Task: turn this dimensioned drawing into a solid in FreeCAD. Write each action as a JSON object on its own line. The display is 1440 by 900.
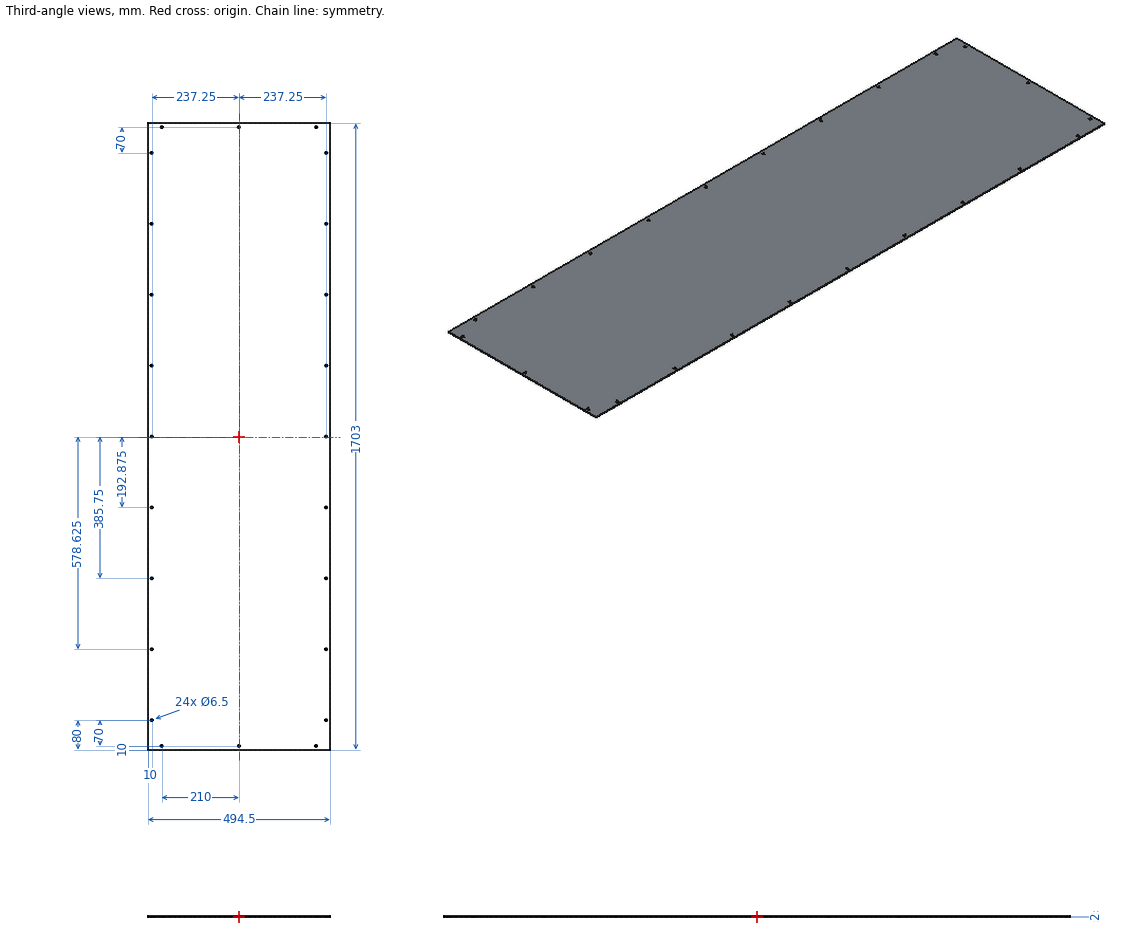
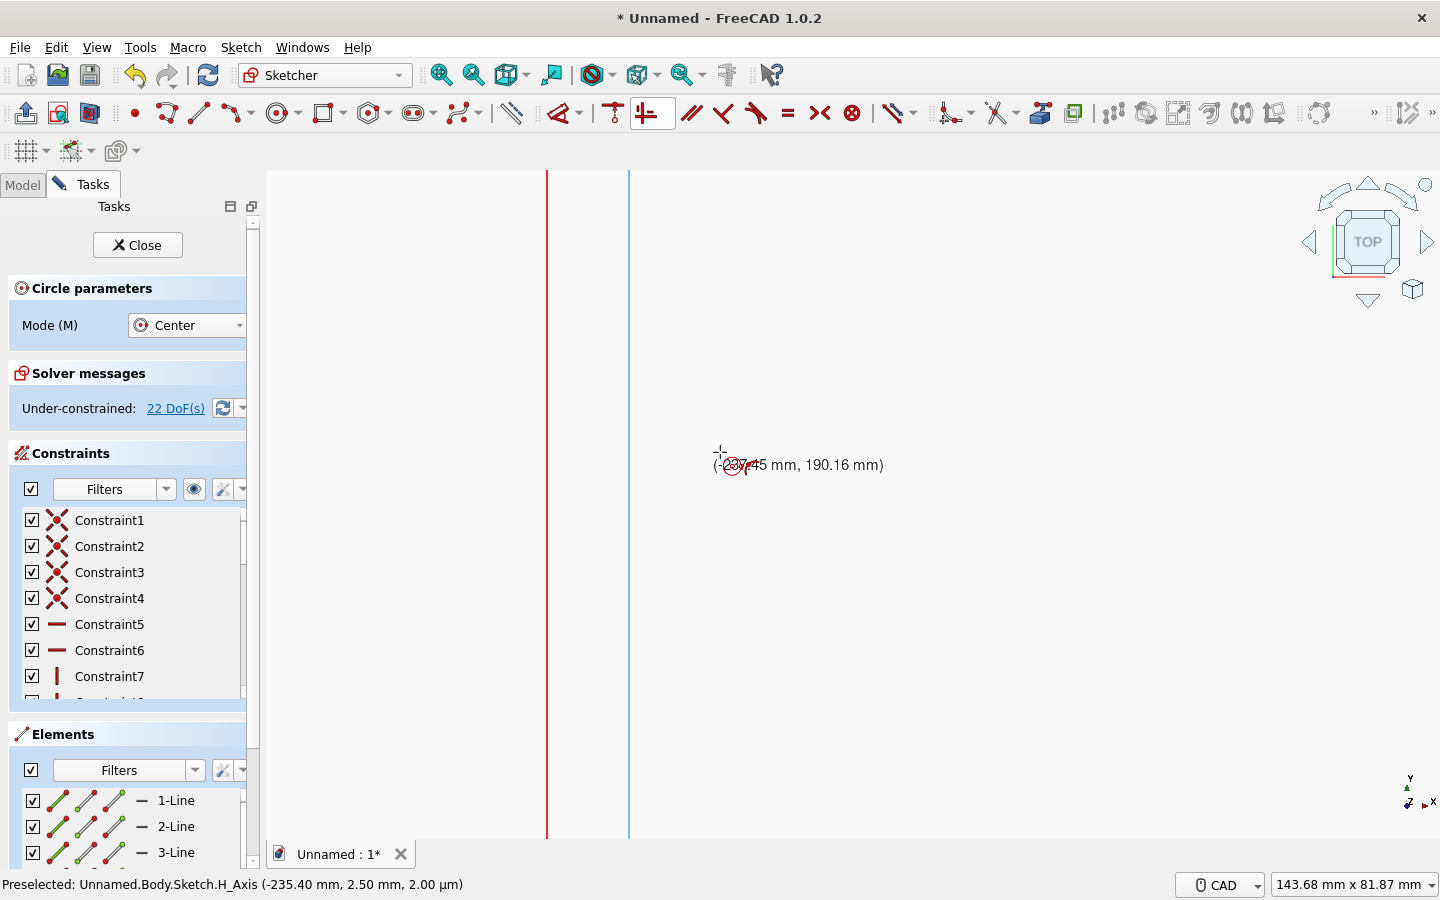
{"action": "scroll", "coordinate": [720, 452], "scroll_direction": "down", "scroll_amount": 17}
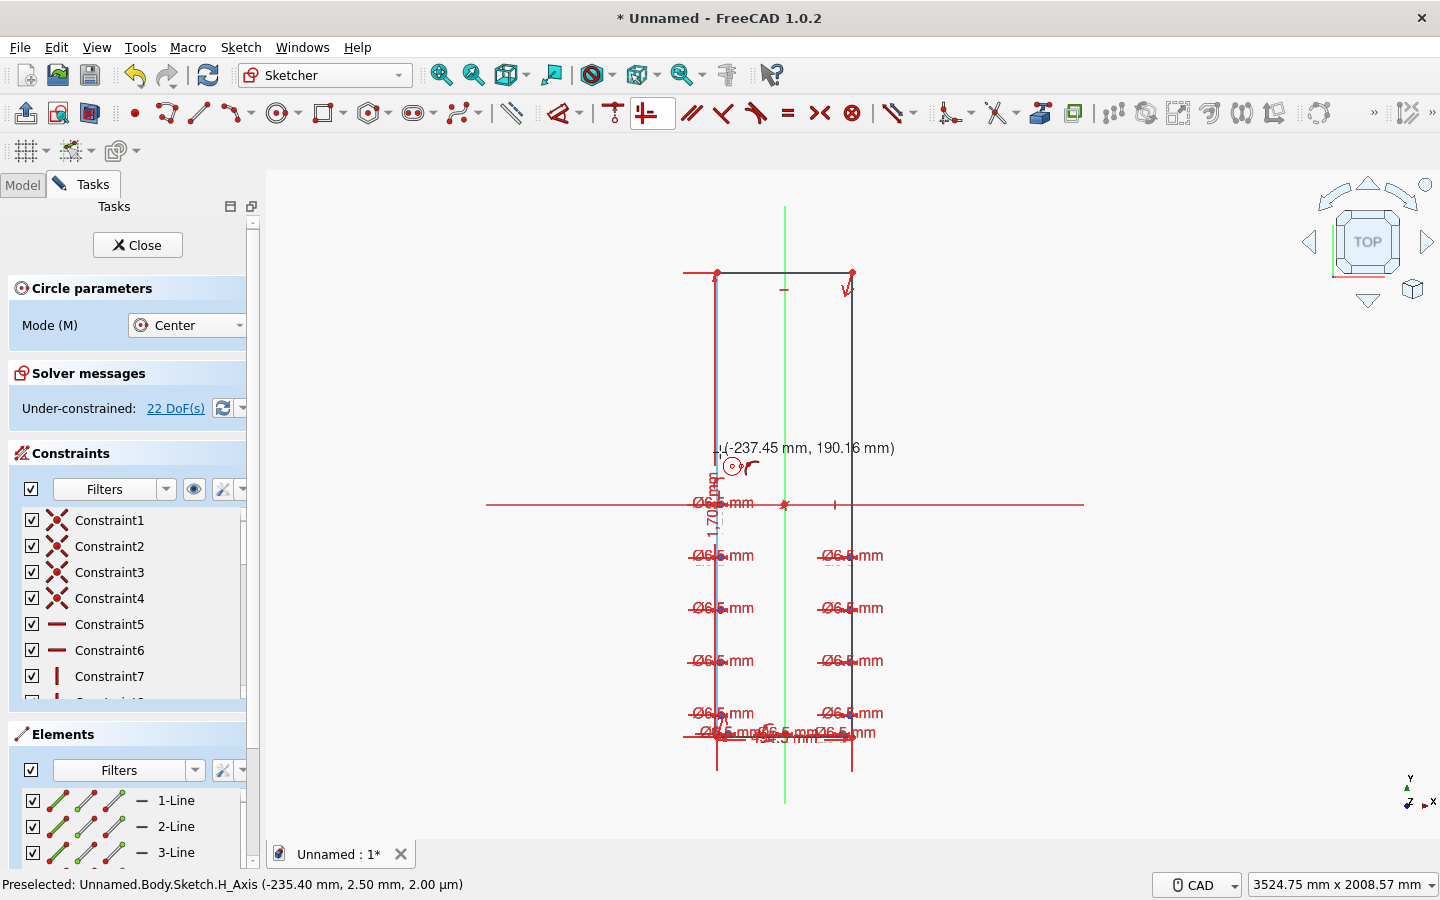
{"action": "scroll", "coordinate": [720, 452], "scroll_direction": "up", "scroll_amount": 9}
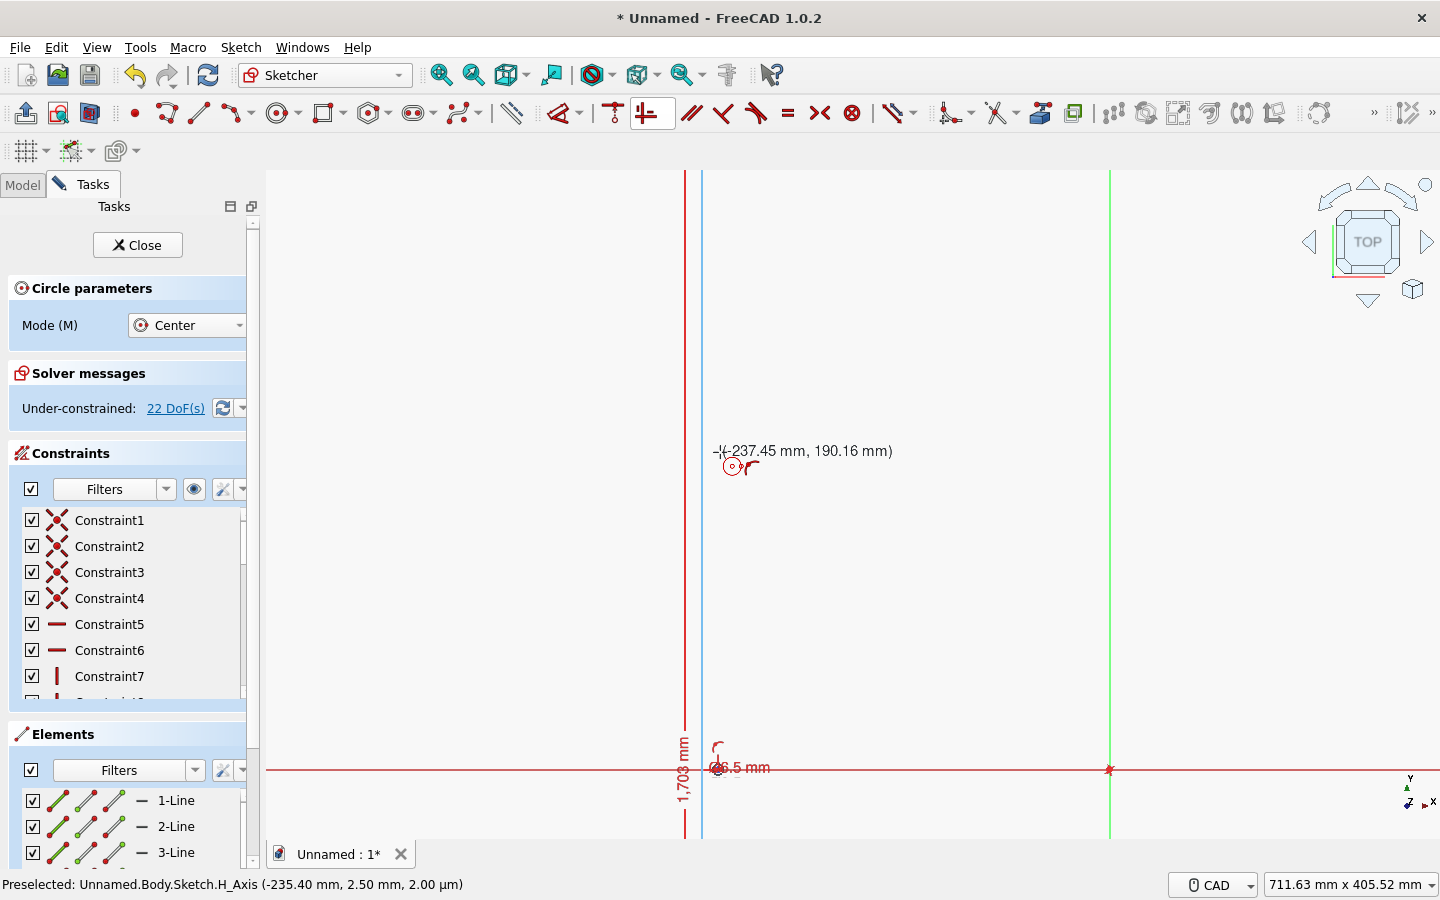
{"action": "left_click", "coordinate": [718, 451]}
{"action": "mouse_move", "coordinate": [722, 448]}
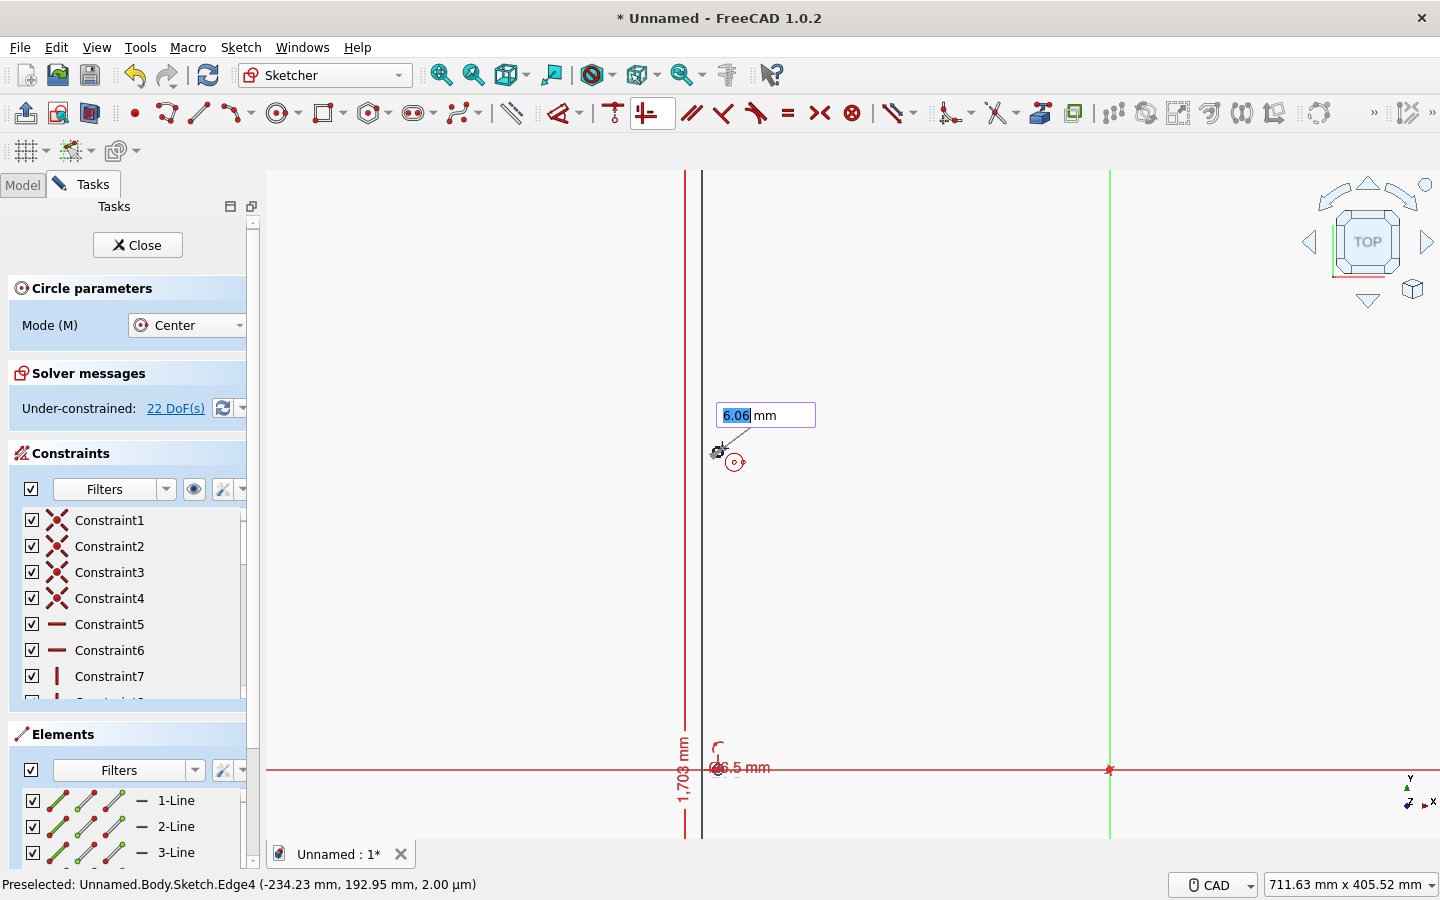
{"action": "type", "text": "6.5"}
{"action": "key", "text": "Return"}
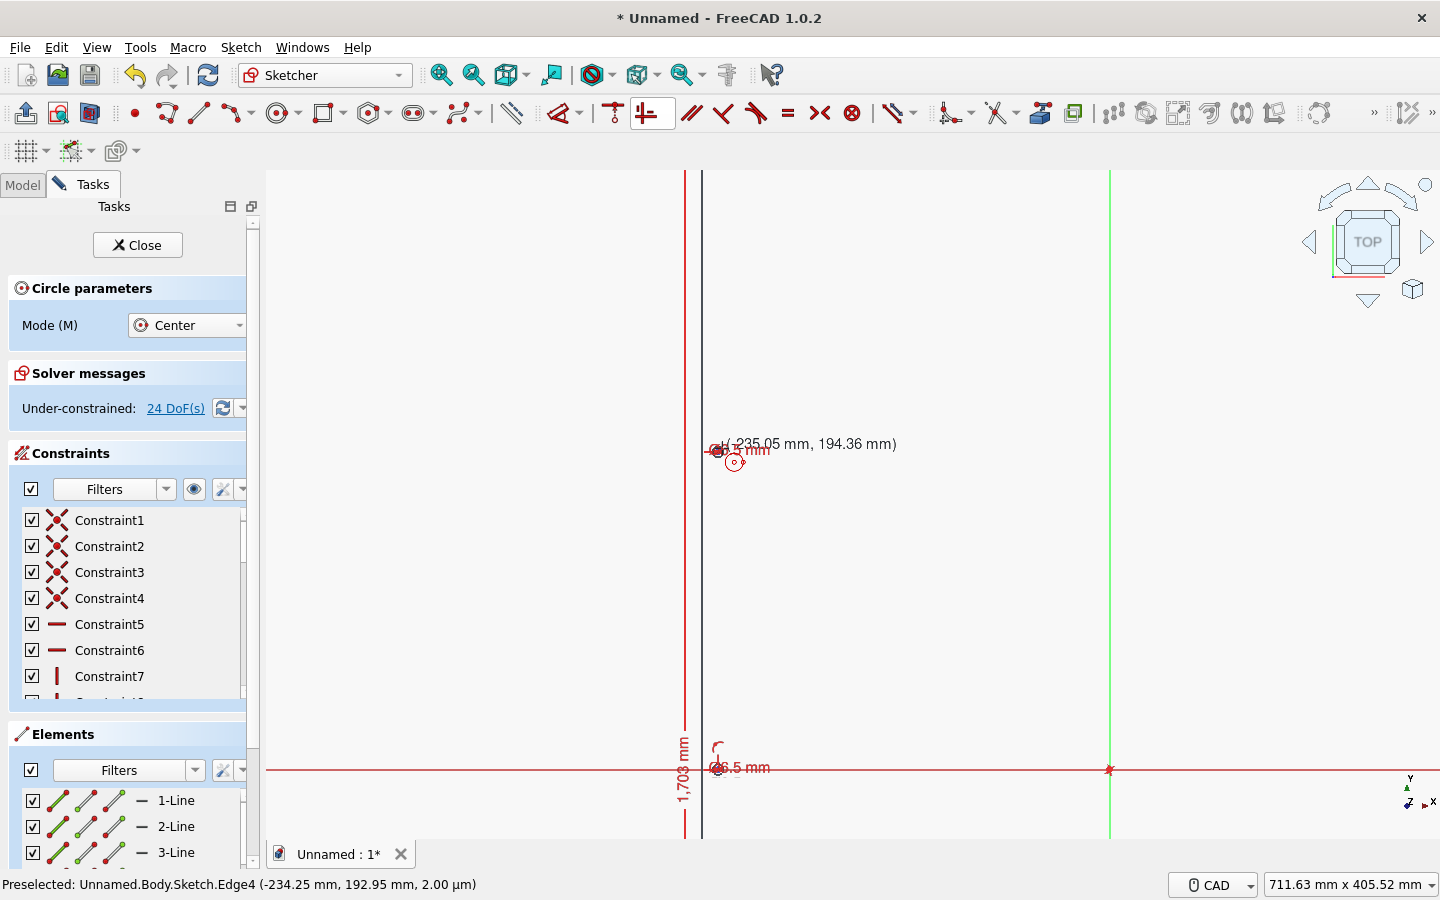
{"action": "scroll", "coordinate": [720, 452], "scroll_direction": "down", "scroll_amount": 9}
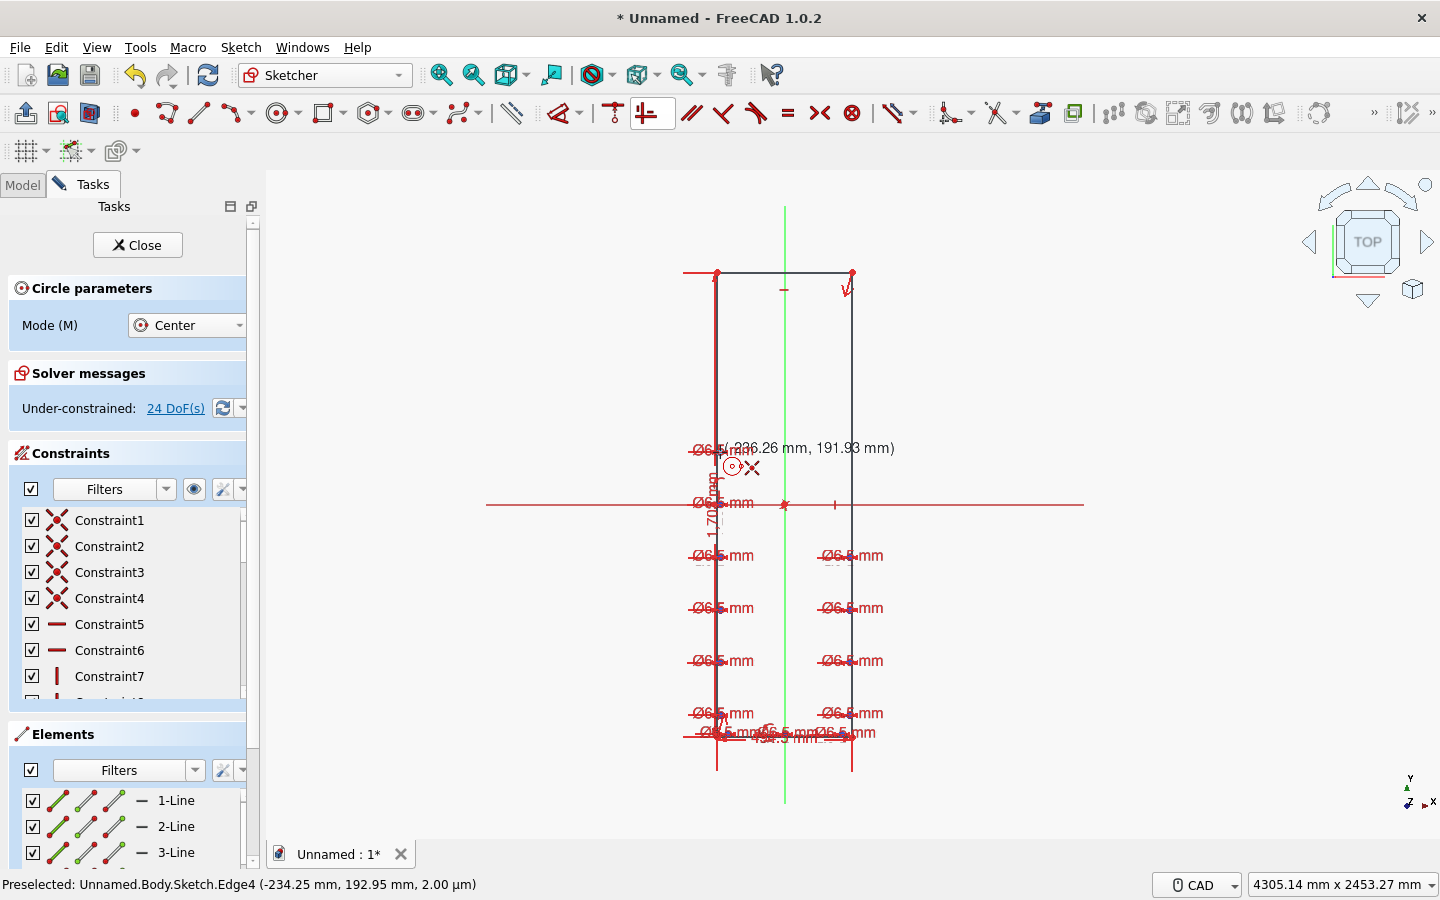
{"action": "scroll", "coordinate": [720, 400], "scroll_direction": "up", "scroll_amount": 17}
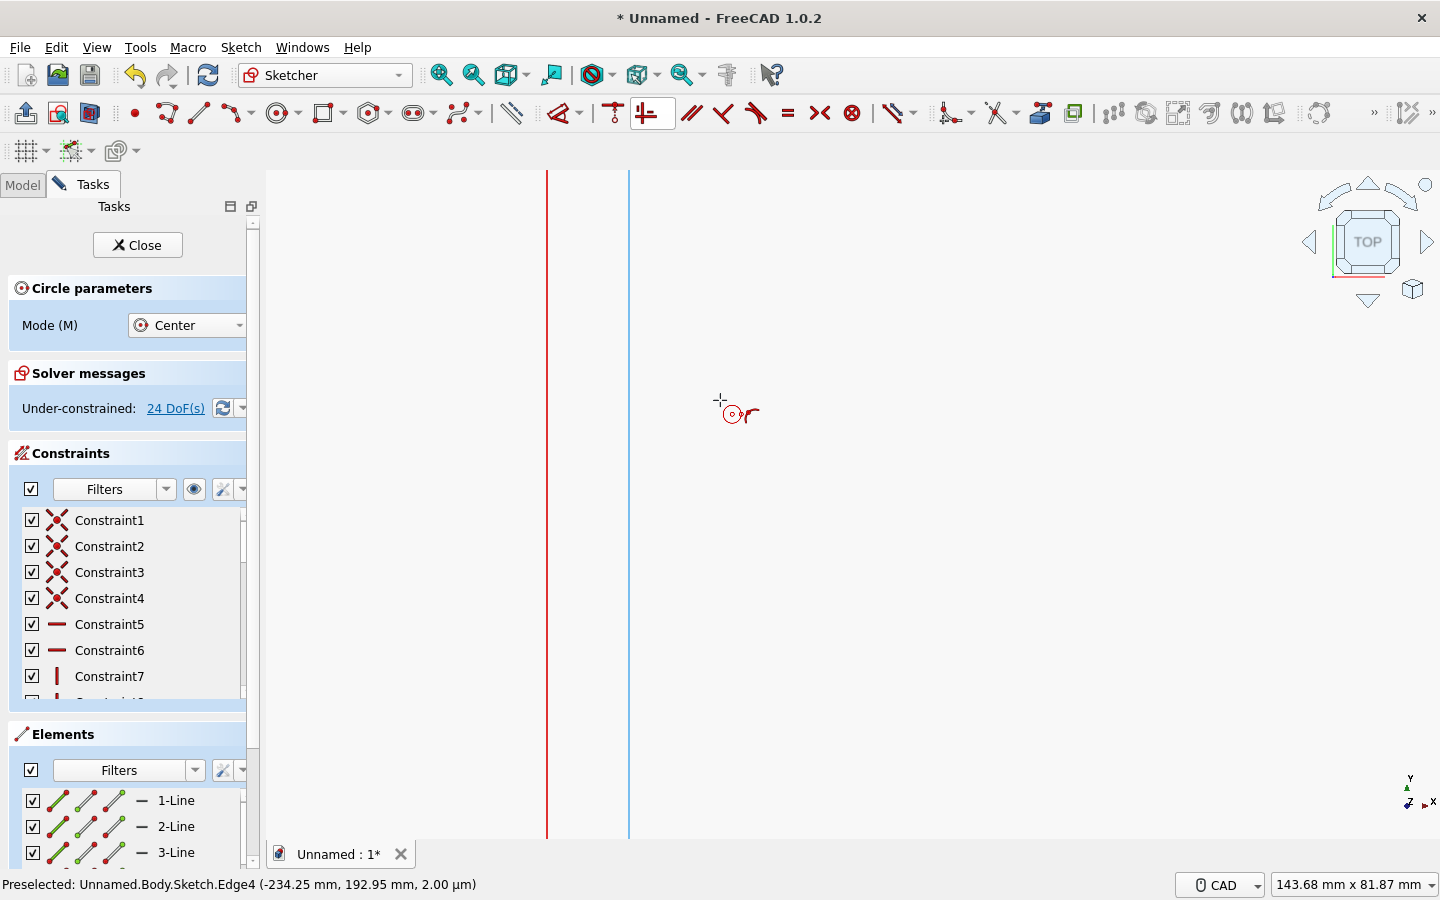
{"action": "scroll", "coordinate": [720, 400], "scroll_direction": "down", "scroll_amount": 17}